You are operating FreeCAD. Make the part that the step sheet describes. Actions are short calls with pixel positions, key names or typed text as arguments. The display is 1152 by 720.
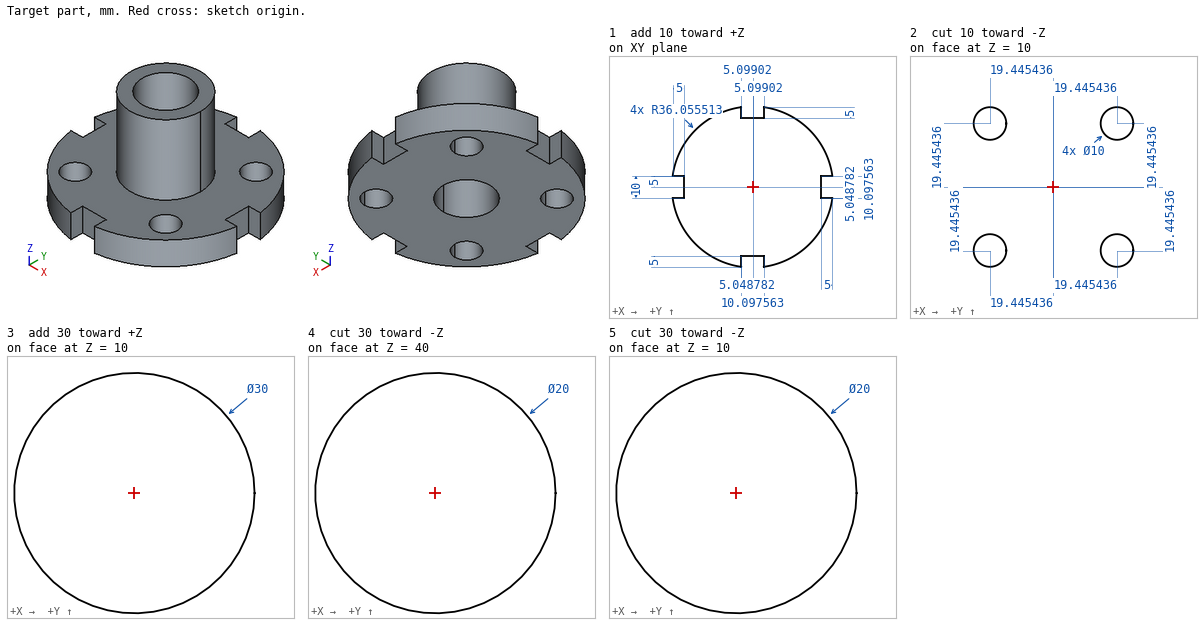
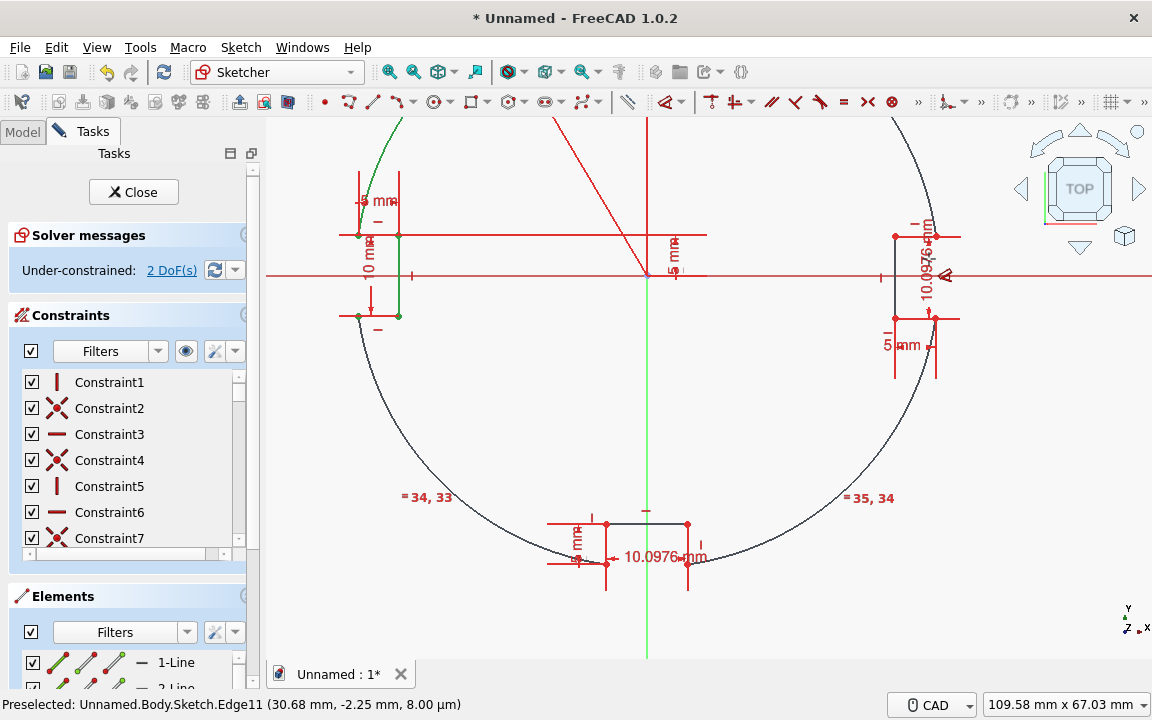
click(606, 564)
click(627, 598)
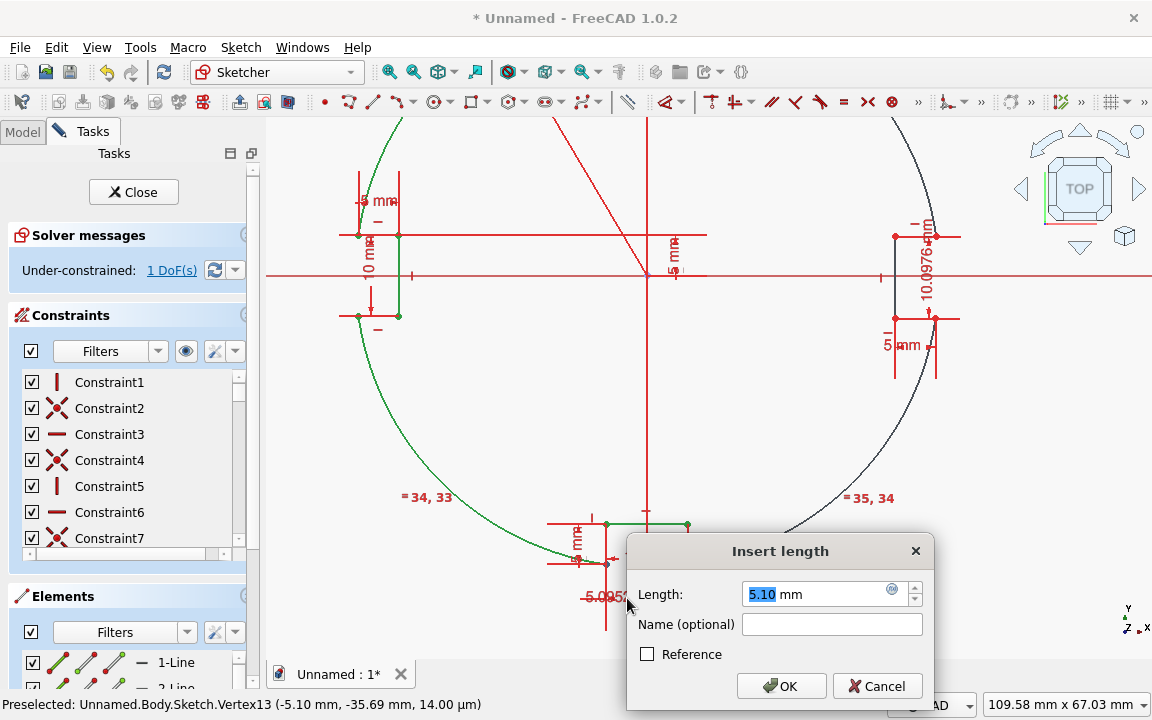
text(5.048782)
key(Return)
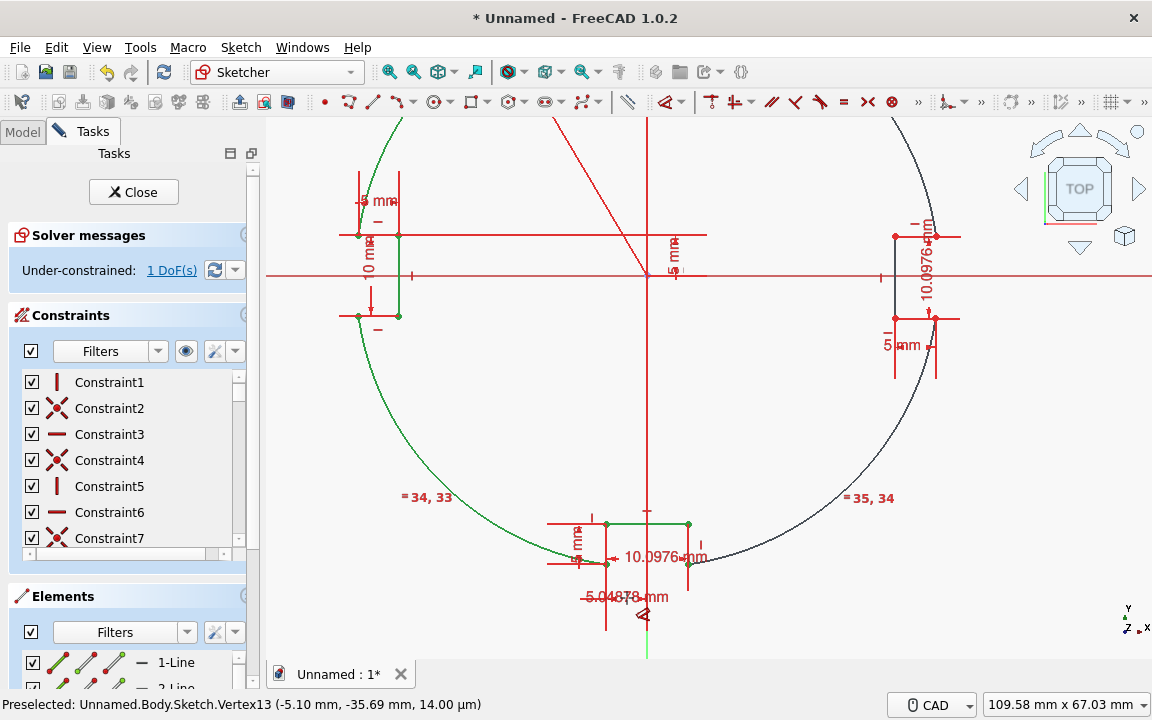
click(936, 319)
click(970, 297)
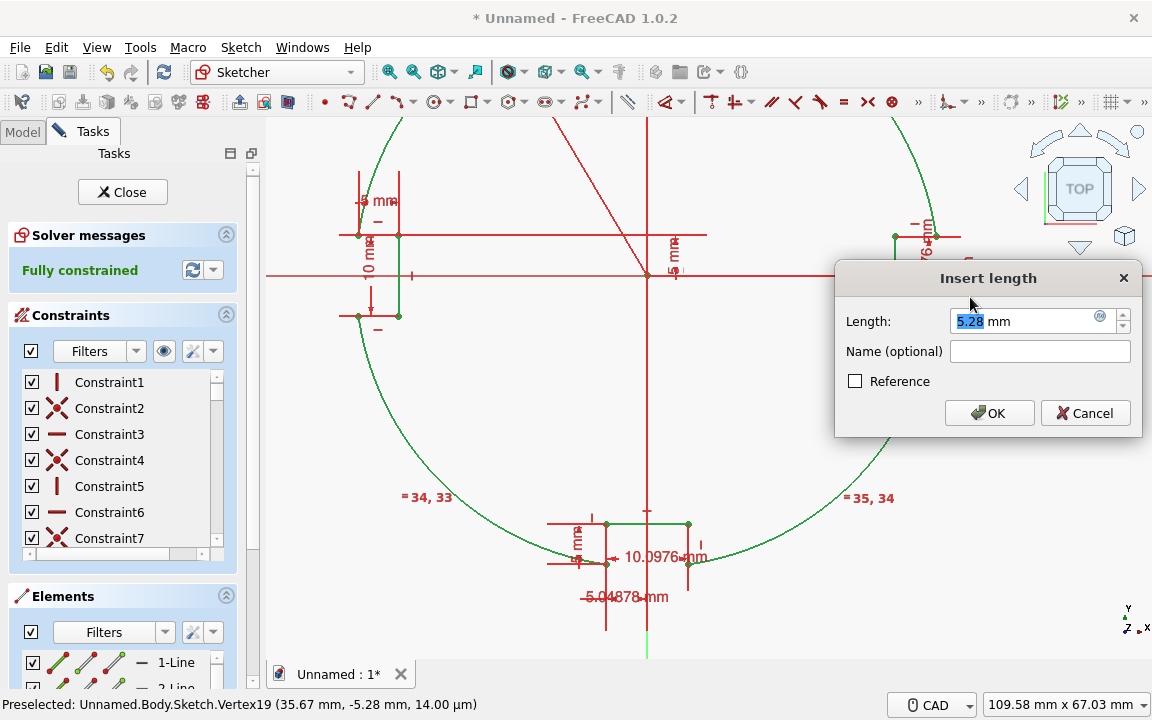
text(5.048782)
key(Return)
key(Escape)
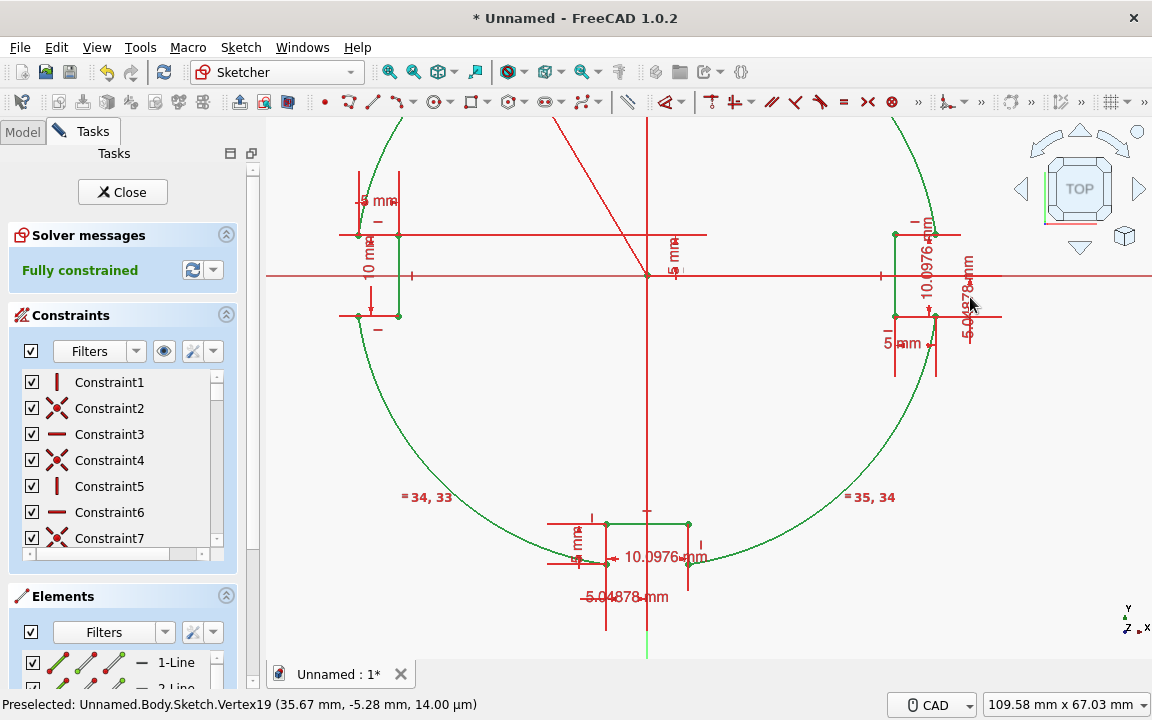
click(123, 192)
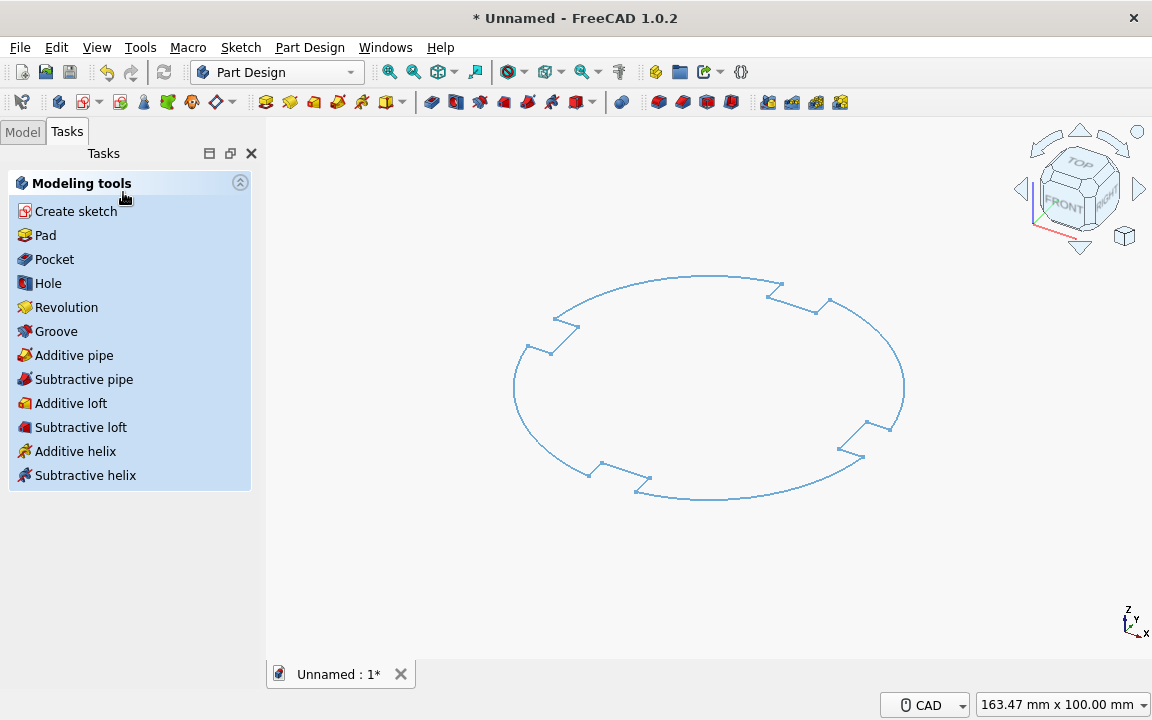
click(266, 102)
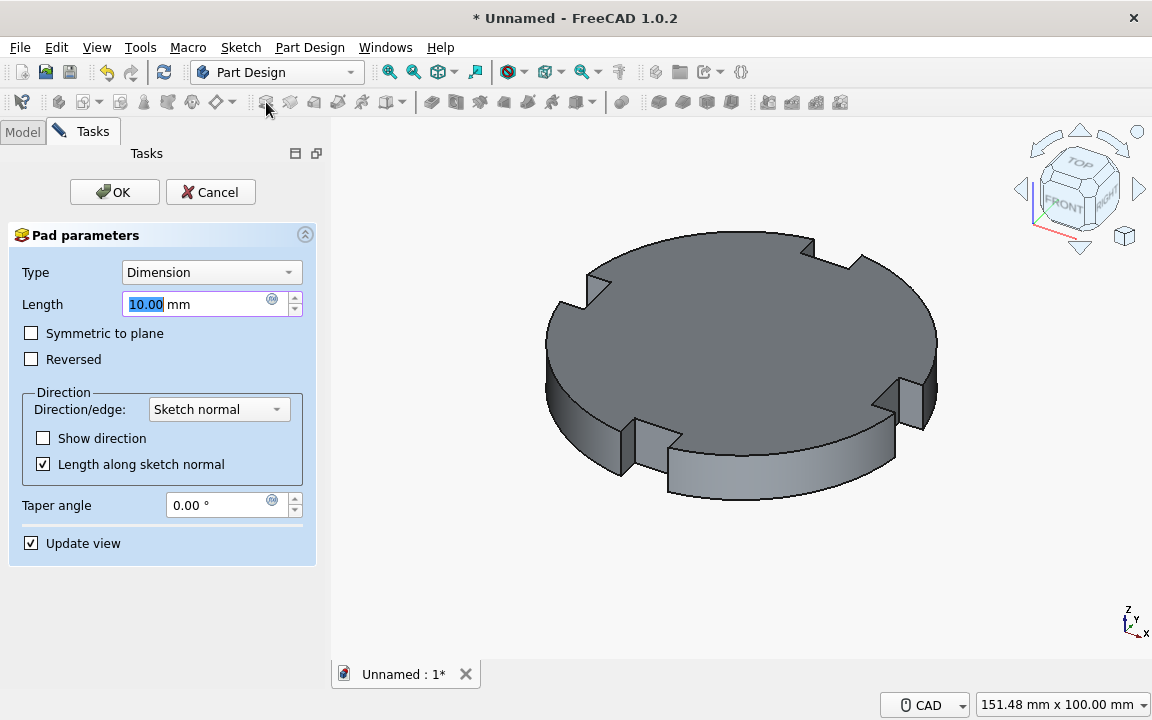
text(10)
key(Tab)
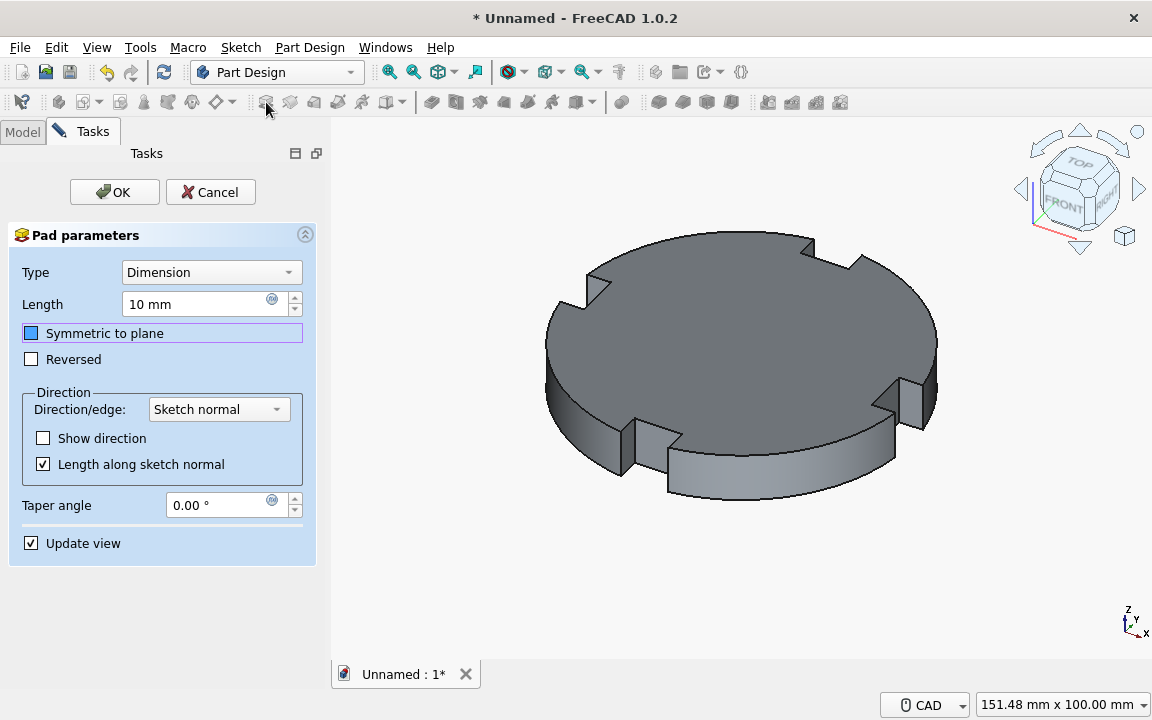
click(115, 192)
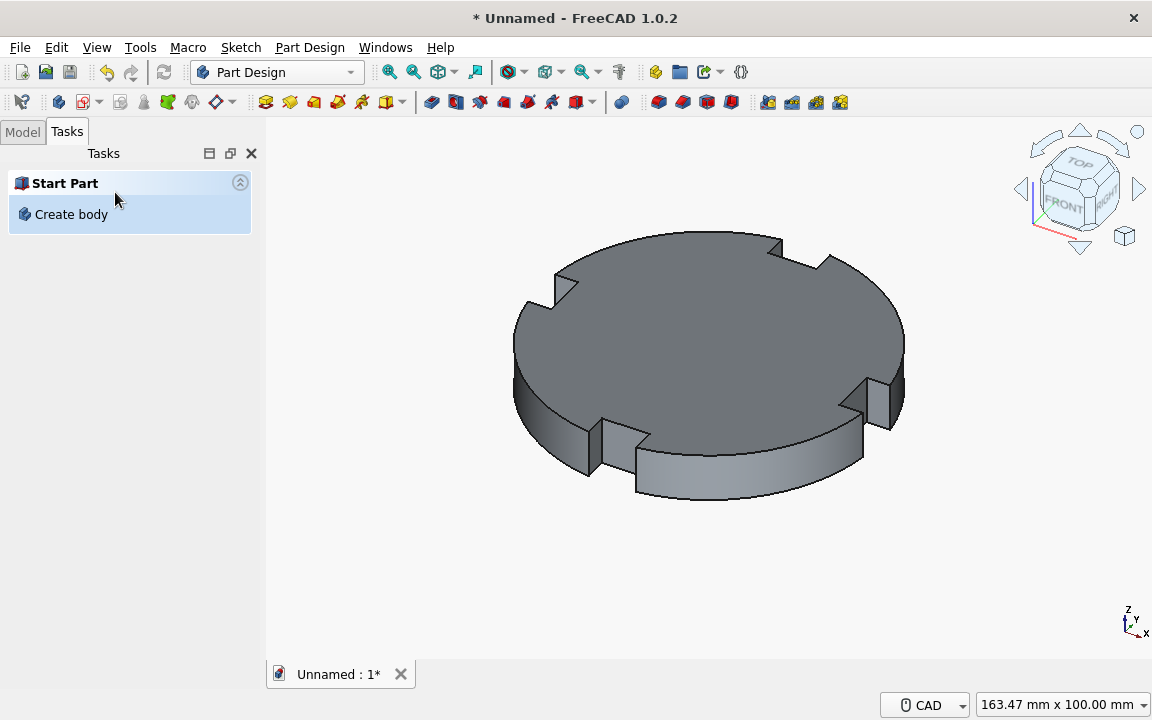
click(709, 343)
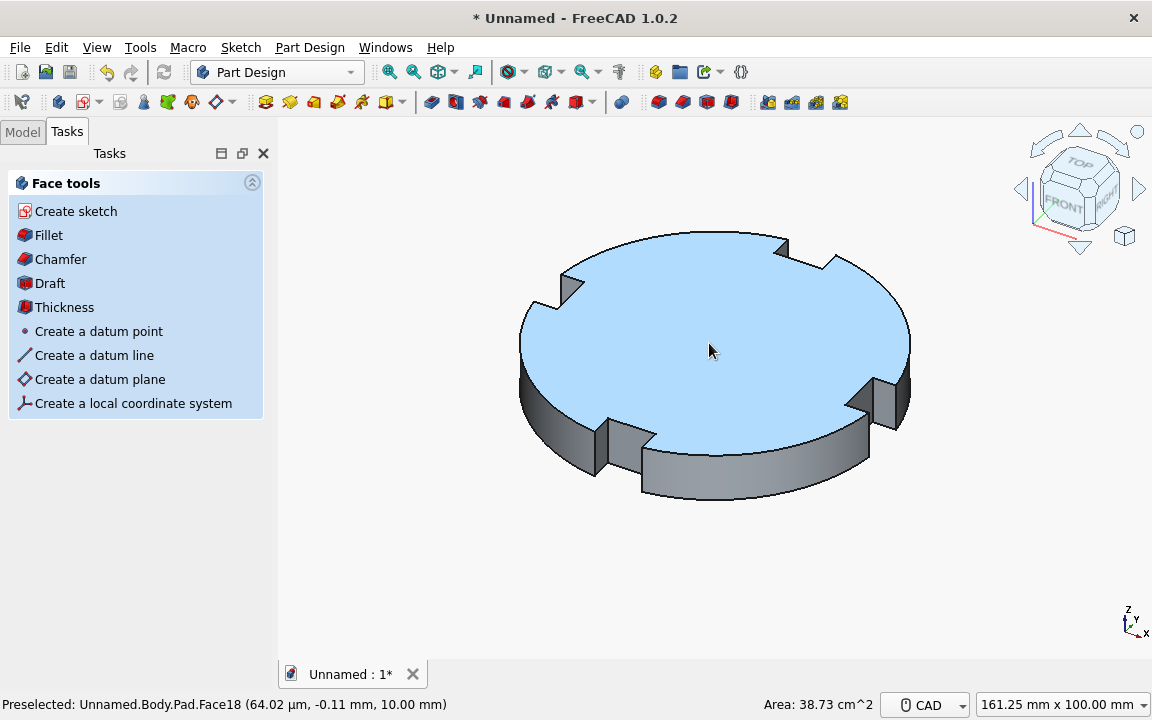
click(84, 102)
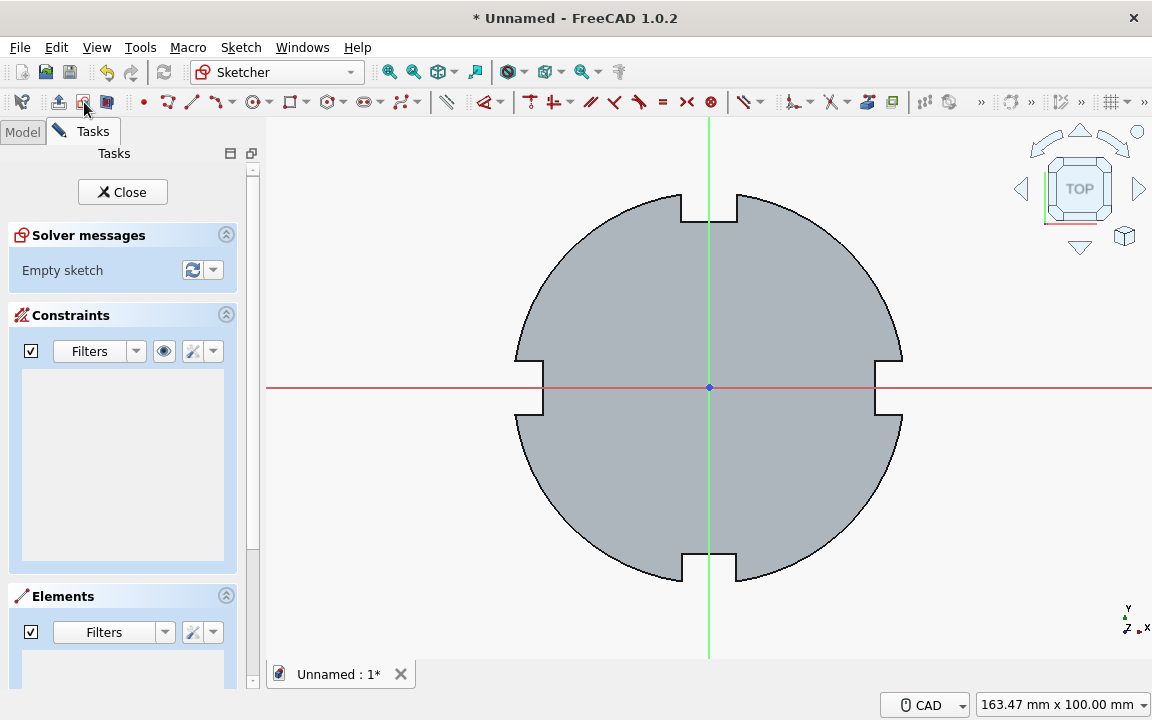
key(g)
key(c)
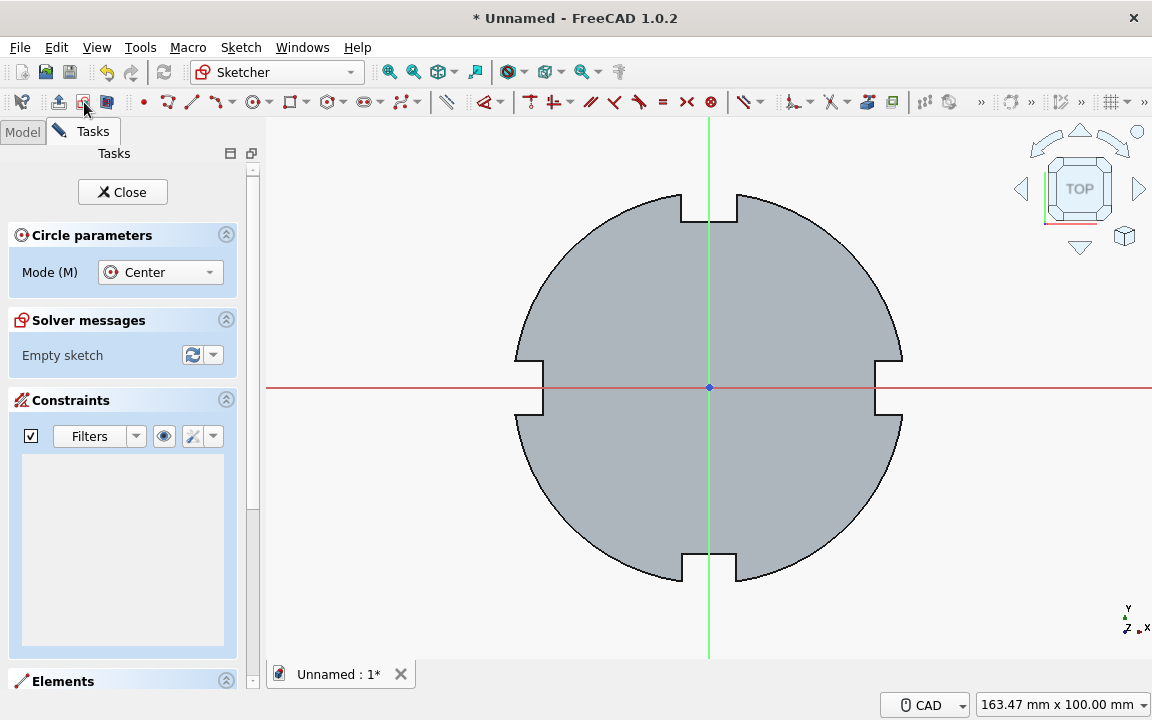
click(814, 283)
move(834, 263)